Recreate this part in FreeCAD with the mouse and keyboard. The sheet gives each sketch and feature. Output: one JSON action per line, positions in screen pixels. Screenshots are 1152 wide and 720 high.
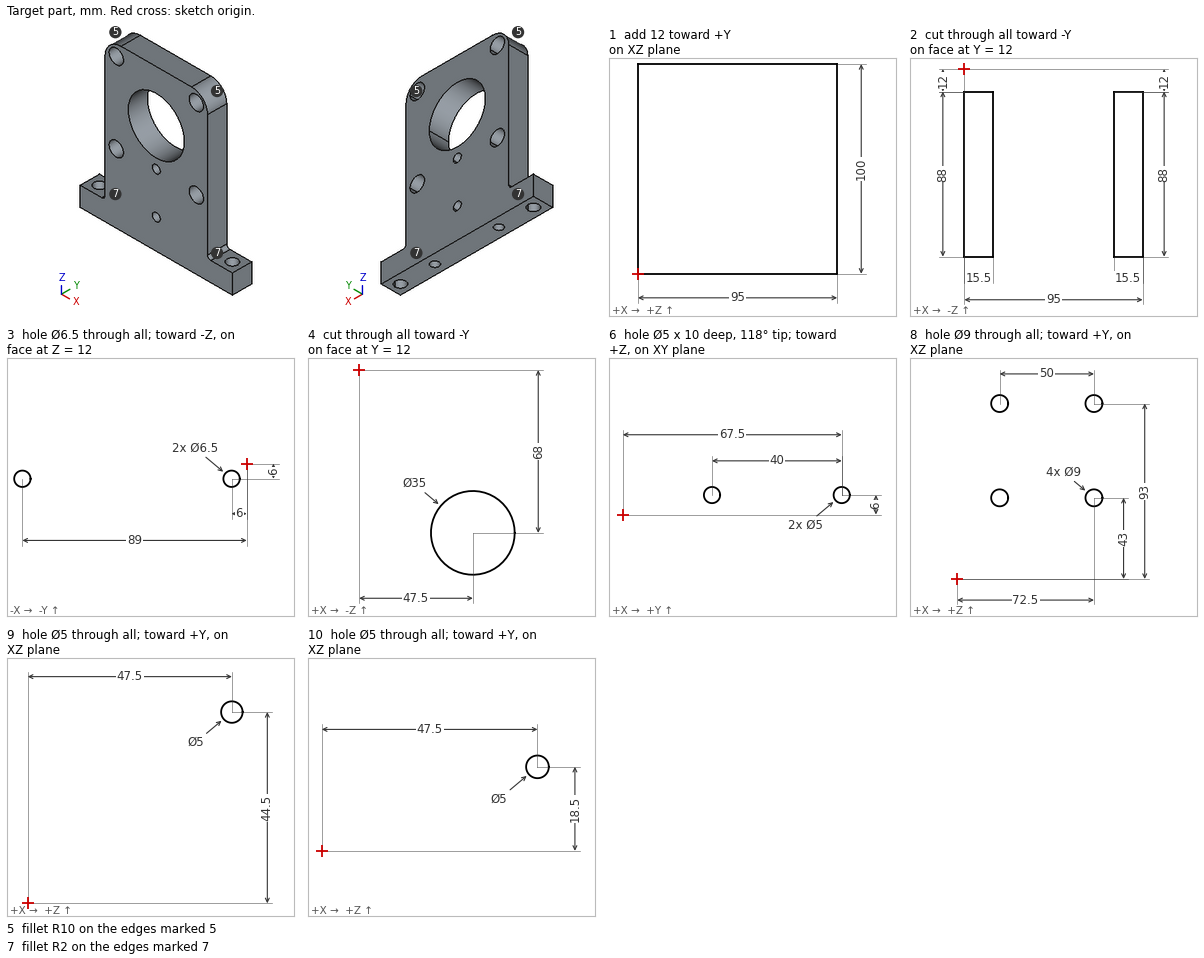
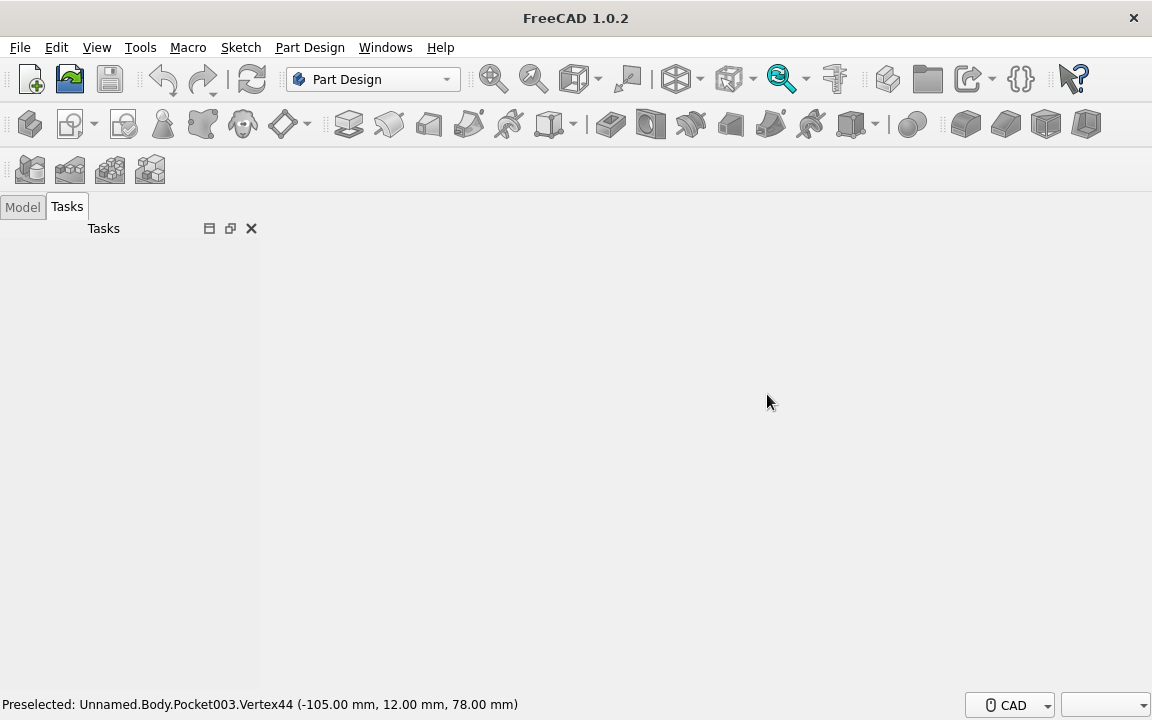
{"action": "left_click", "coordinate": [30, 80]}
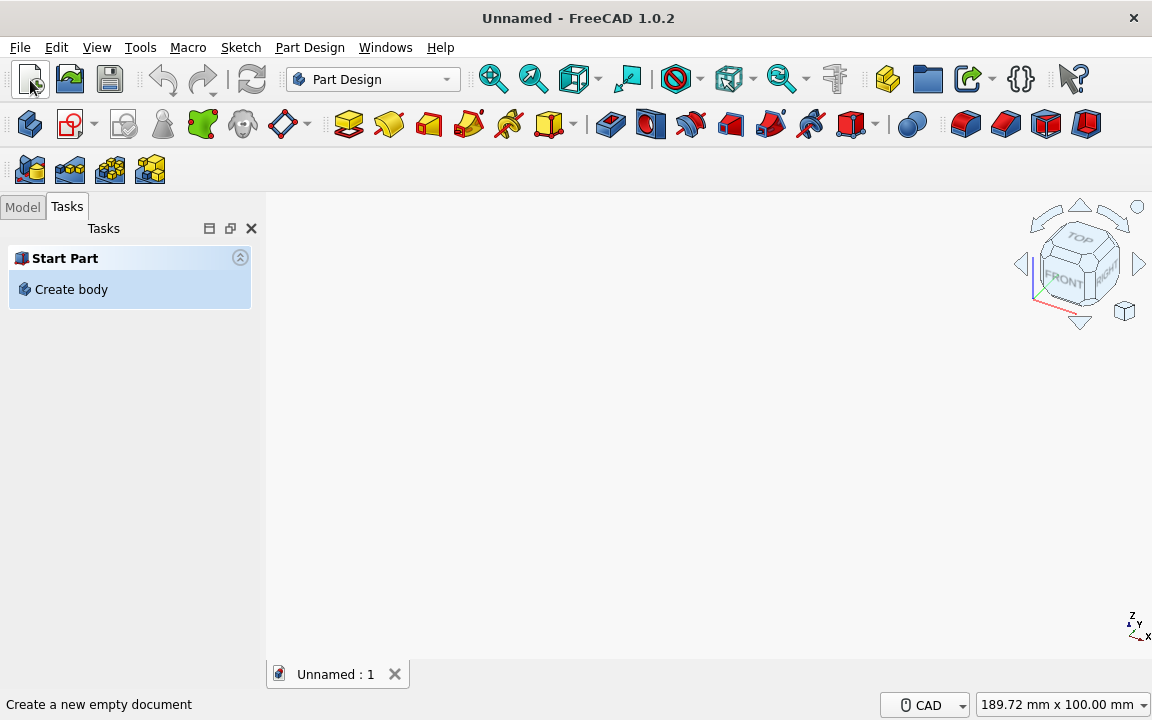
{"action": "left_click", "coordinate": [70, 124]}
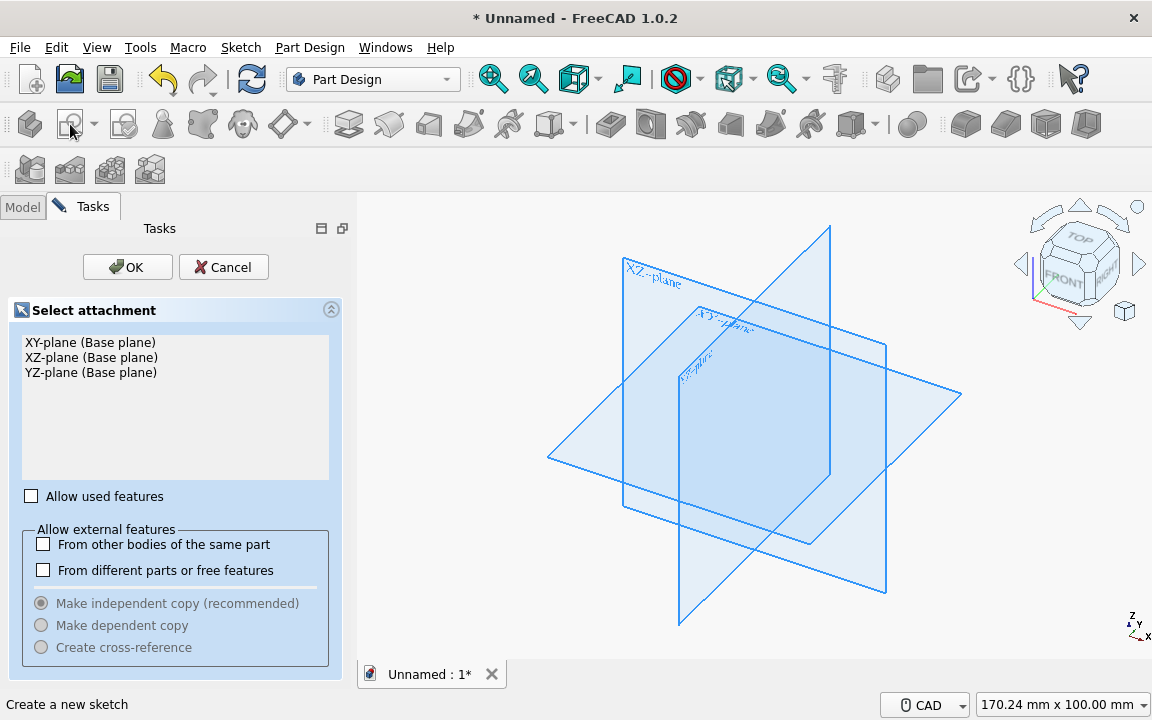
{"action": "left_click", "coordinate": [82, 358]}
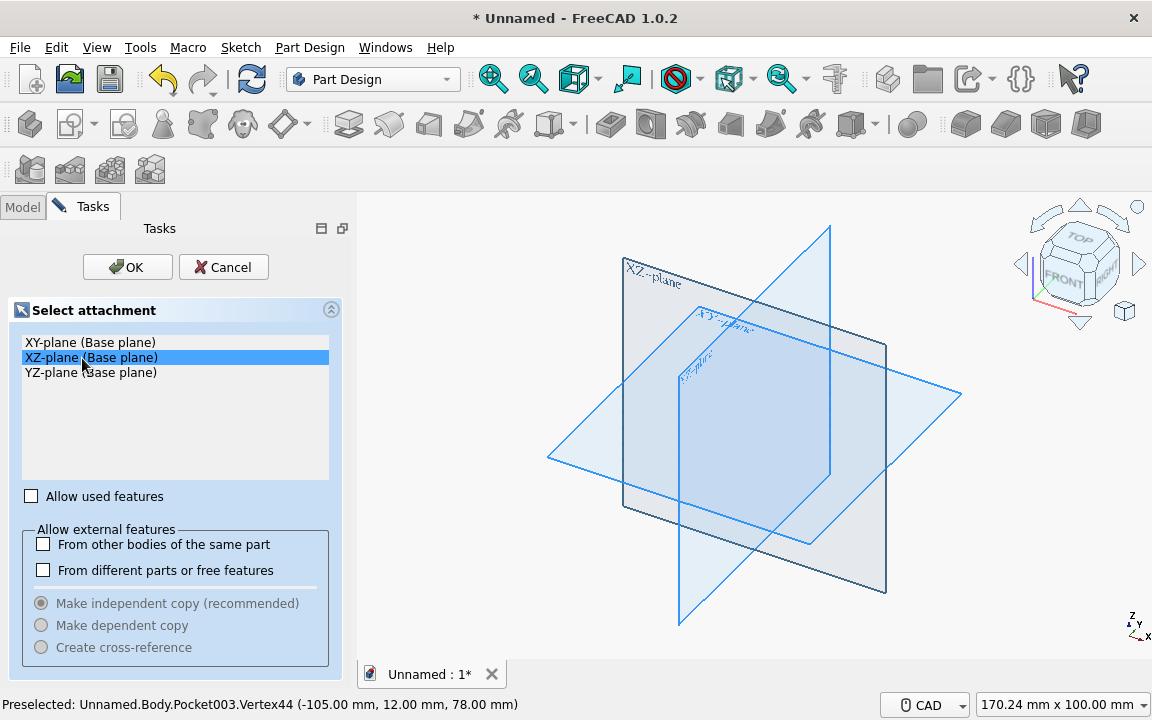
{"action": "left_click", "coordinate": [128, 267]}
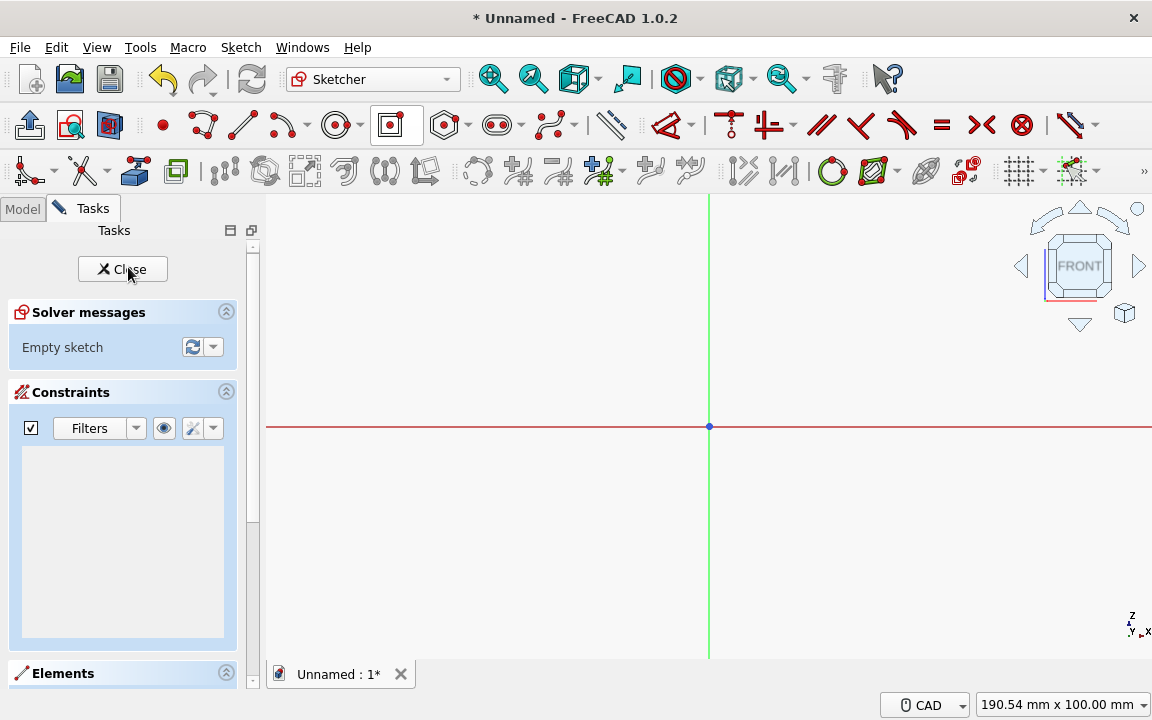
{"action": "scroll", "coordinate": [294, 631], "scroll_direction": "down", "scroll_amount": 3}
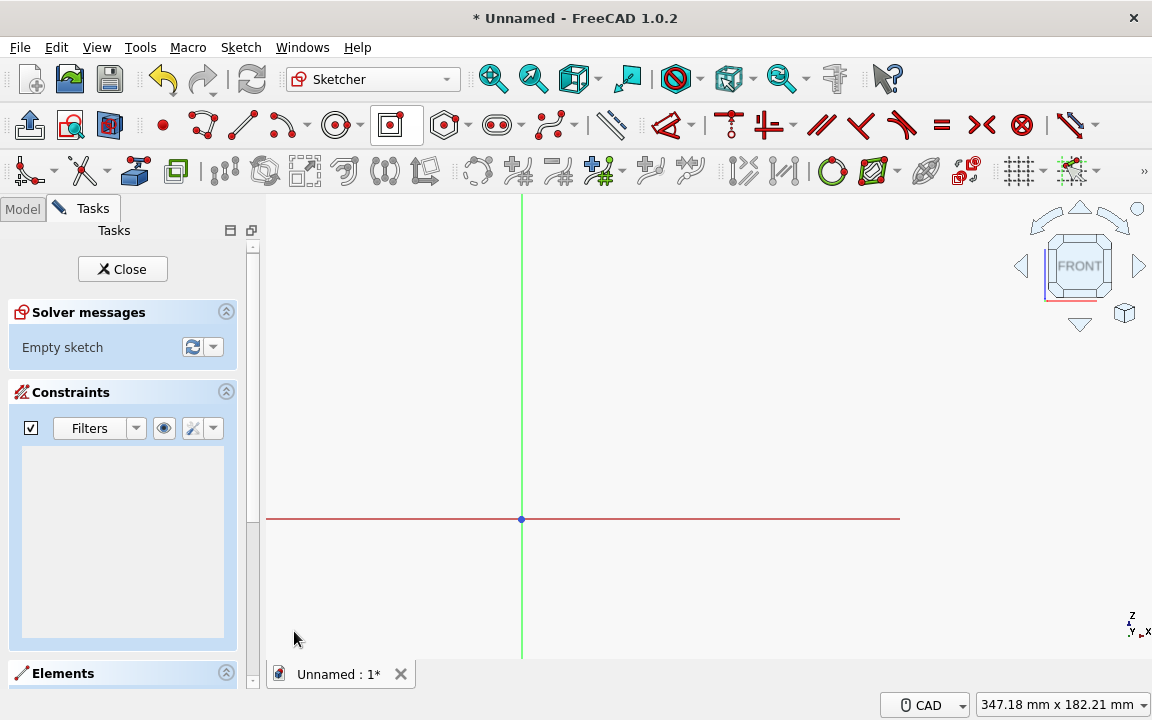
{"action": "key", "text": "g r"}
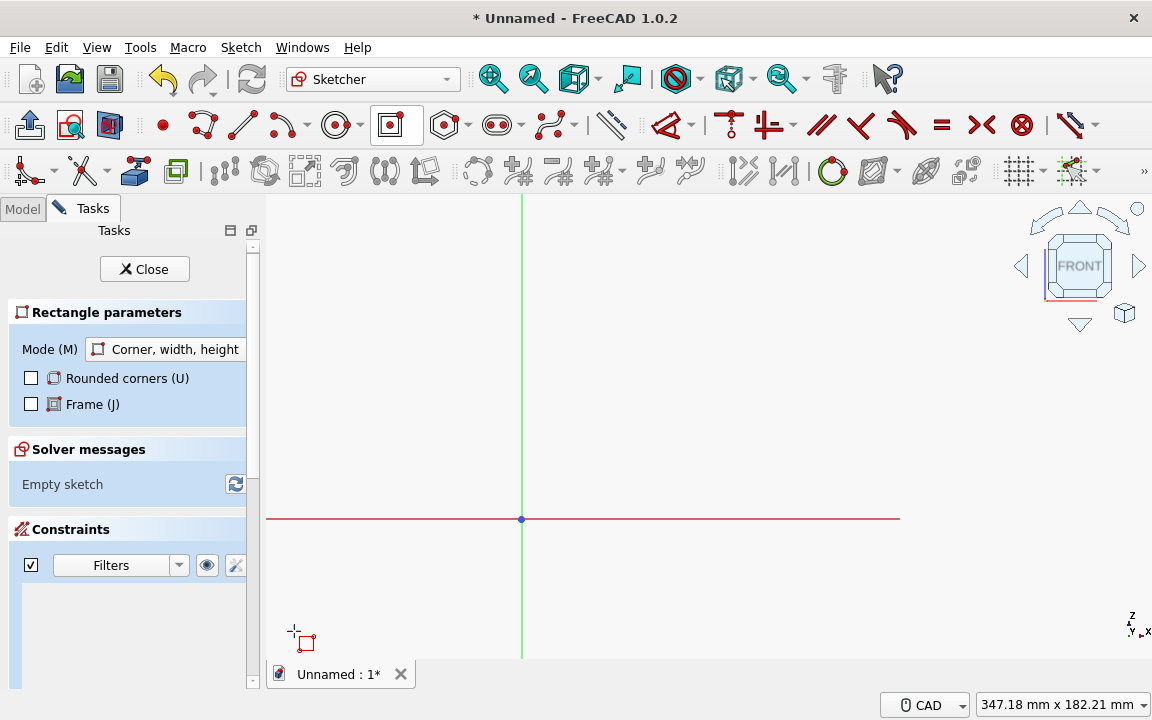
{"action": "left_click", "coordinate": [522, 519]}
{"action": "left_click", "coordinate": [764, 264]}
{"action": "key", "text": "Escape"}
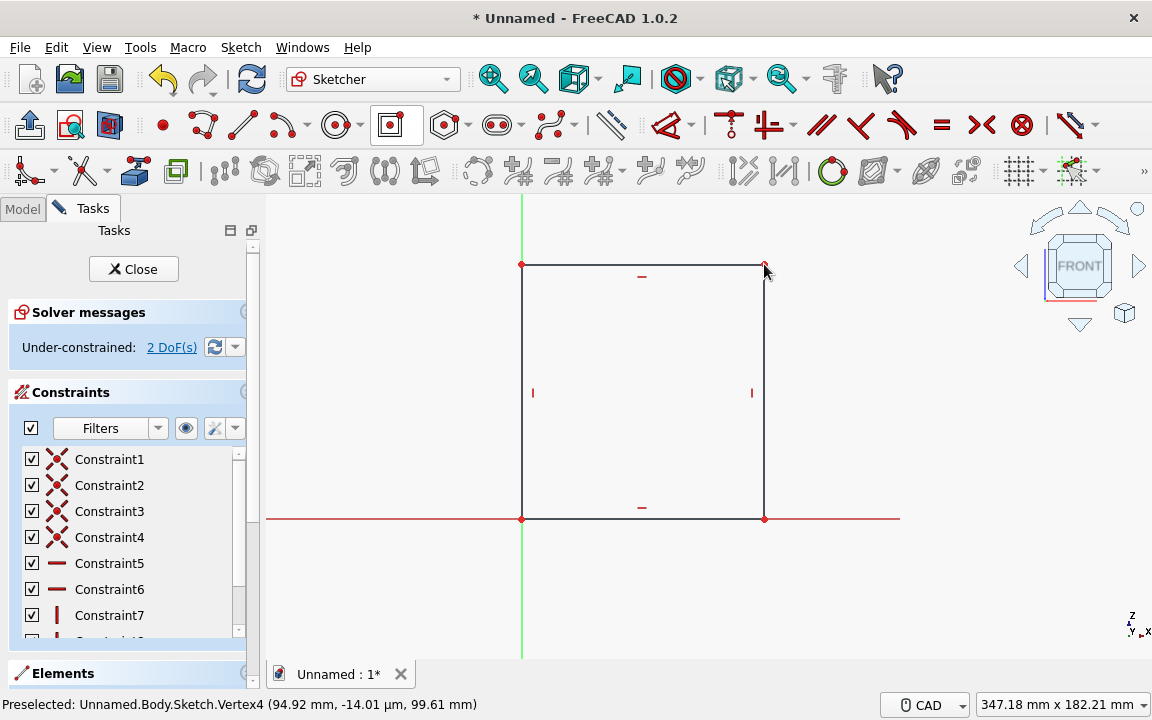
{"action": "left_click", "coordinate": [666, 126]}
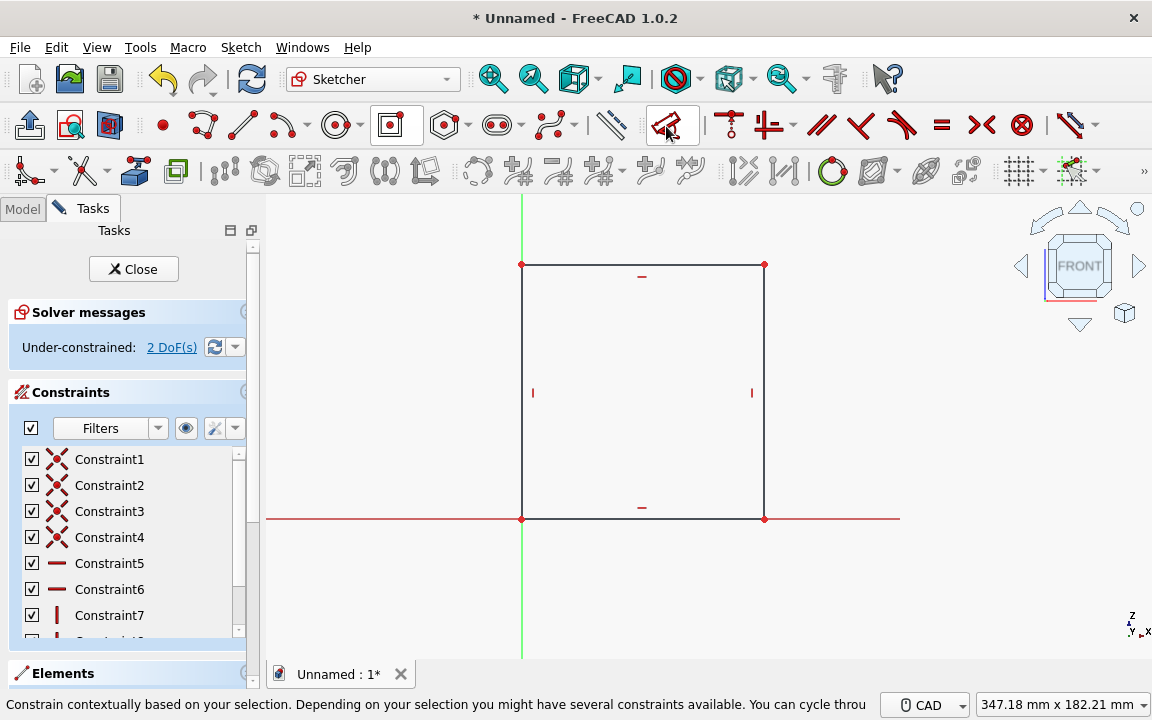
{"action": "left_click", "coordinate": [594, 519]}
{"action": "left_click", "coordinate": [643, 553]}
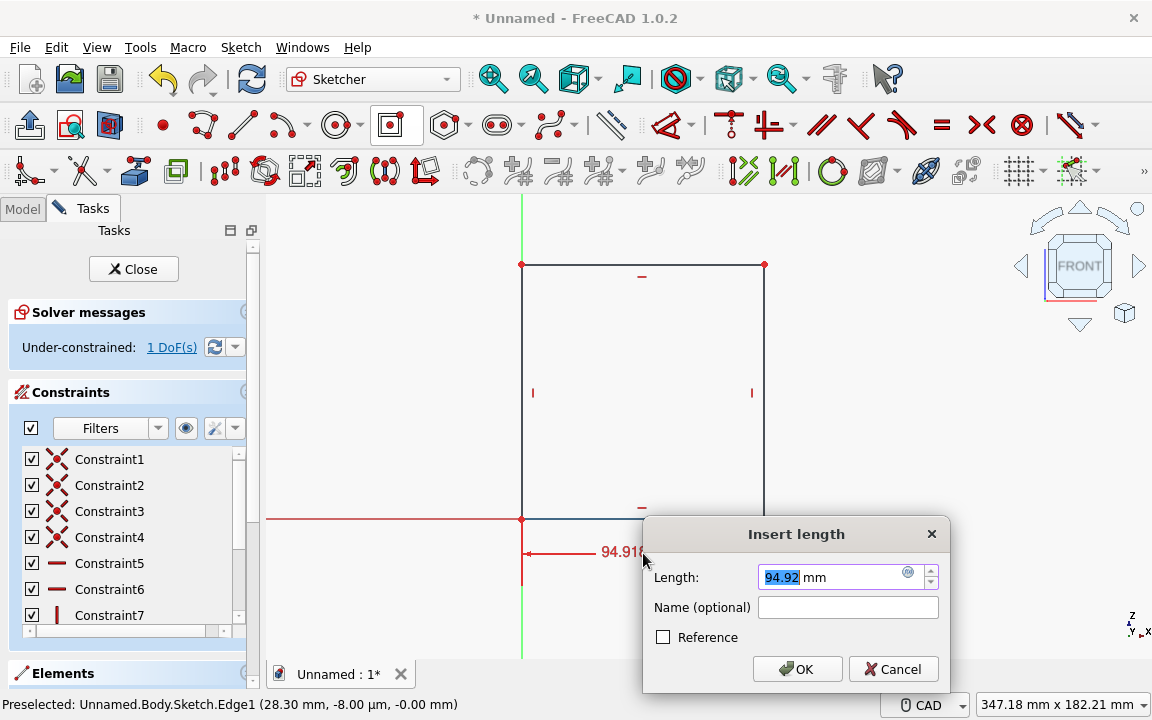
{"action": "type", "text": "95"}
{"action": "key", "text": "Return"}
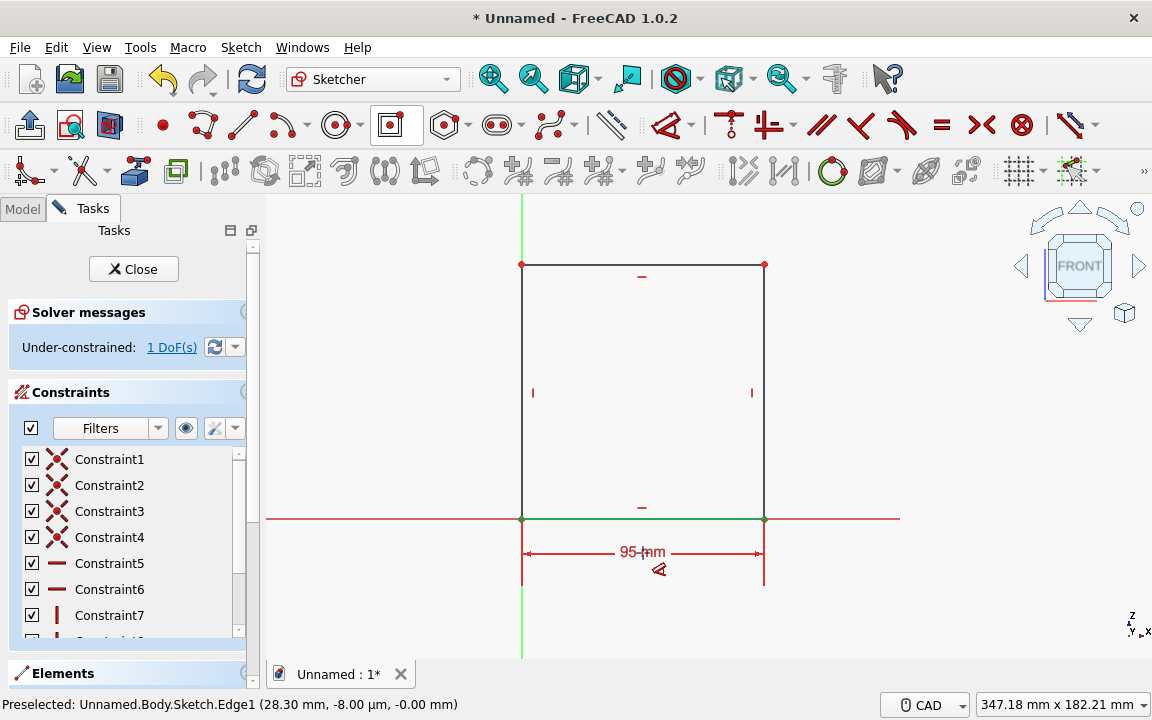
{"action": "left_click", "coordinate": [764, 443]}
{"action": "left_click", "coordinate": [798, 392]}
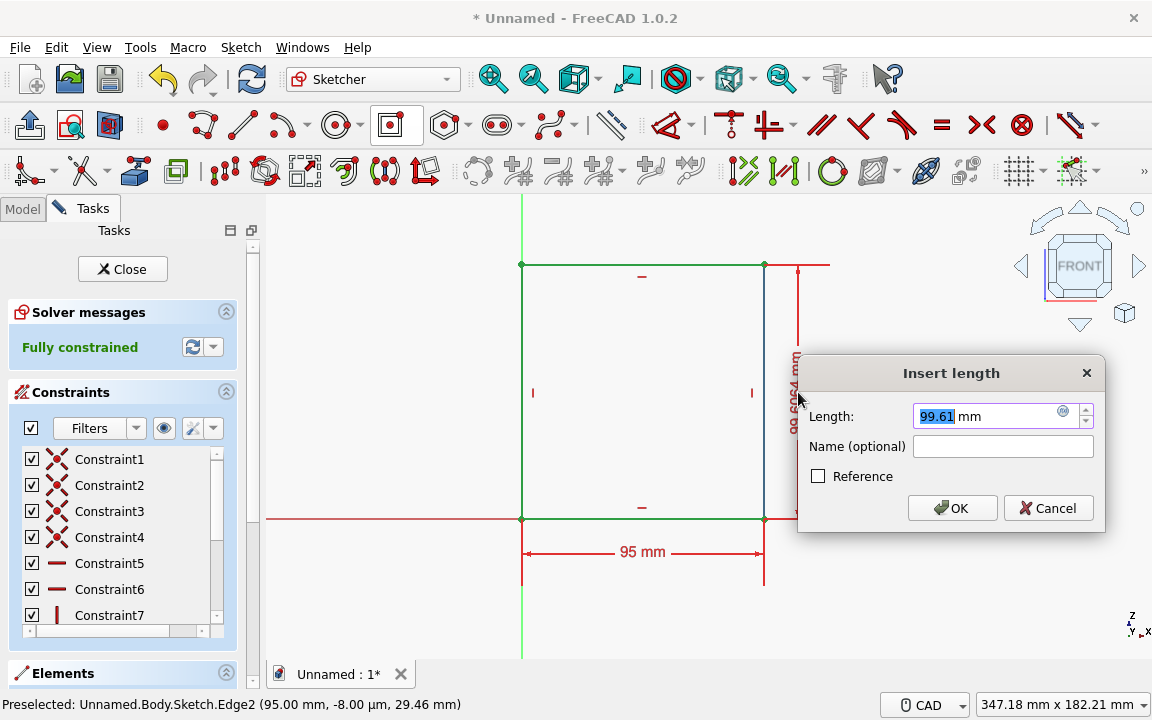
{"action": "type", "text": "100"}
{"action": "key", "text": "Return"}
{"action": "key", "text": "Escape"}